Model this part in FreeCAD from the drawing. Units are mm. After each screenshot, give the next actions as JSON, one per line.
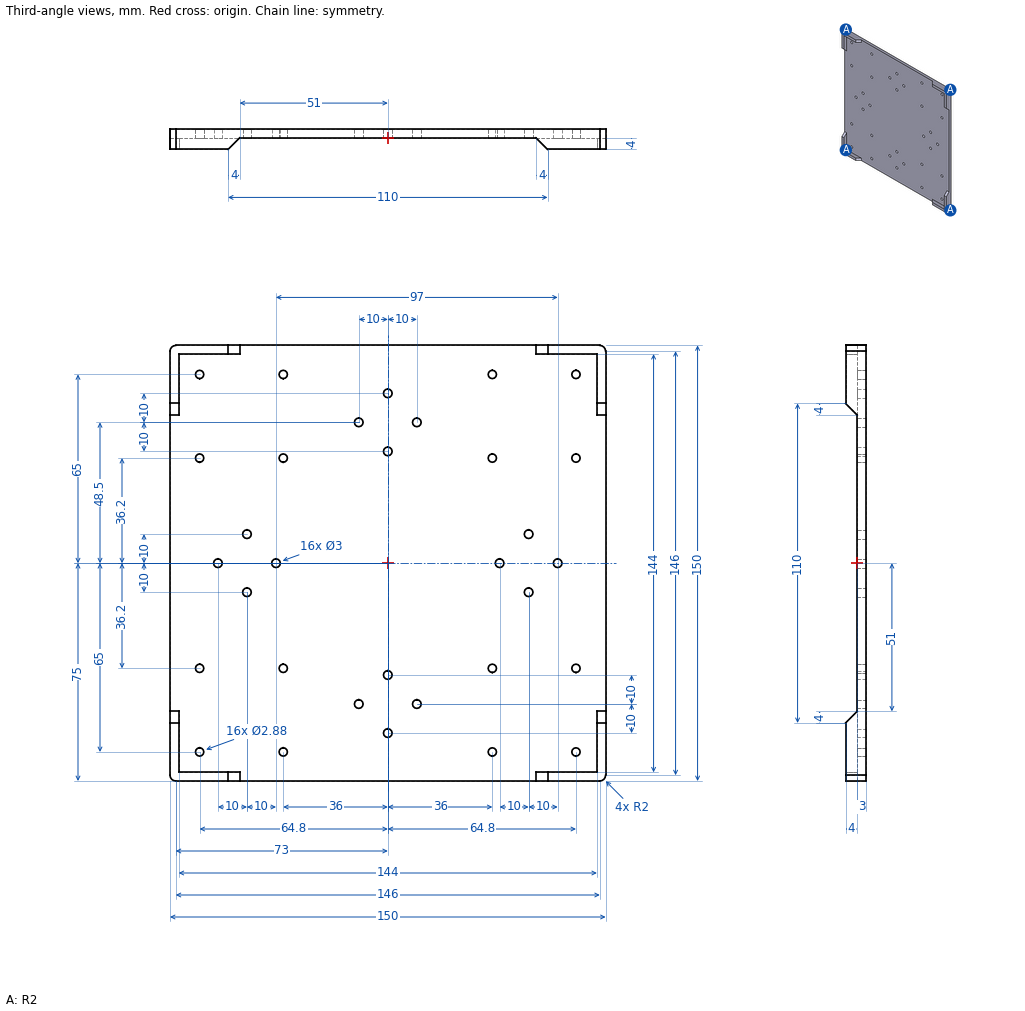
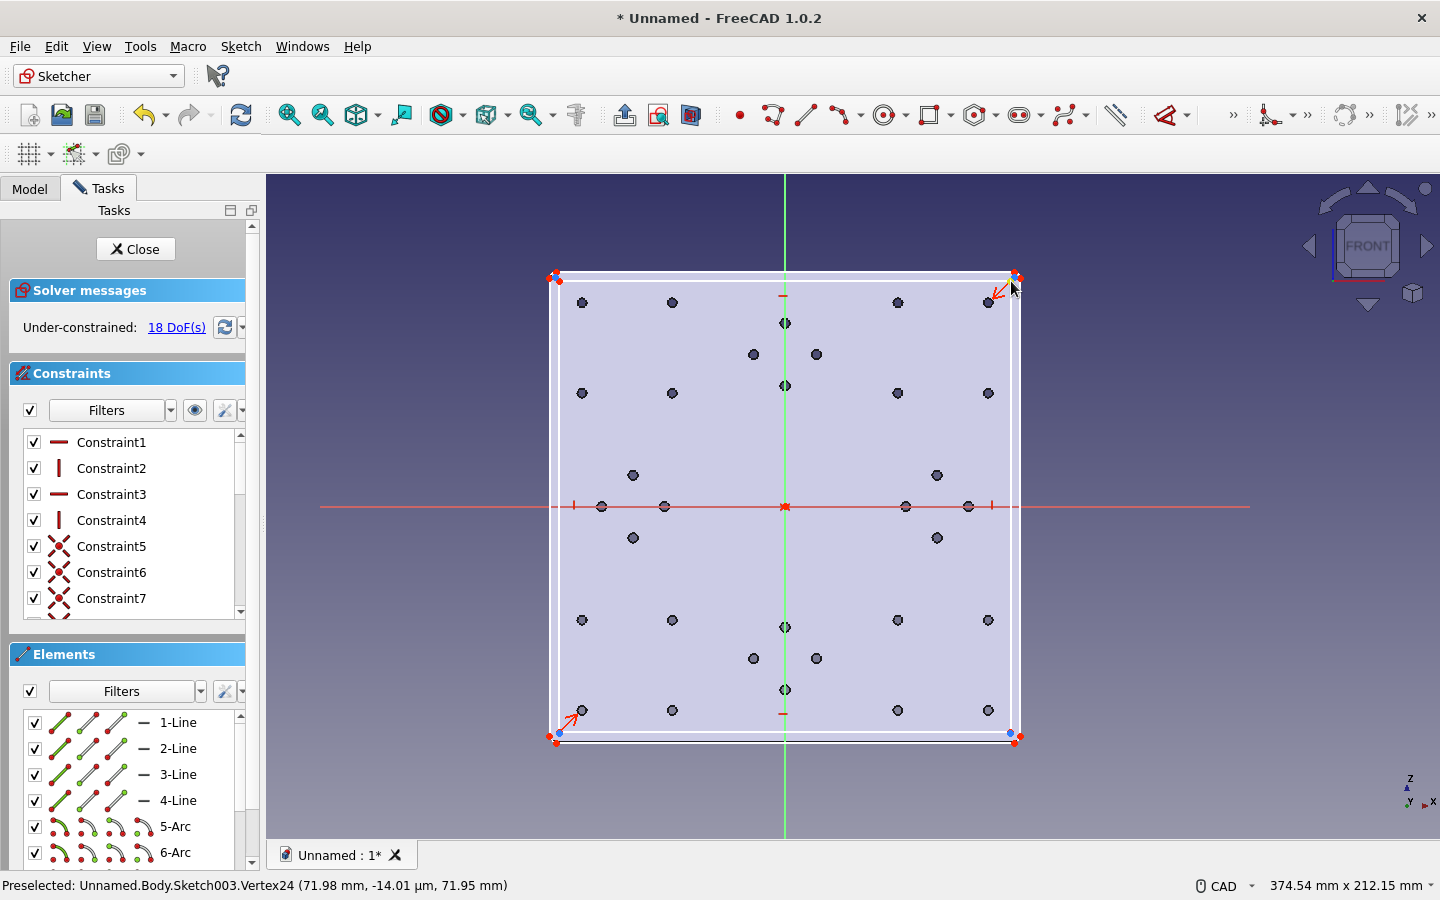
{"action": "scroll", "coordinate": [694, 743], "scroll_direction": "up", "scroll_amount": 2}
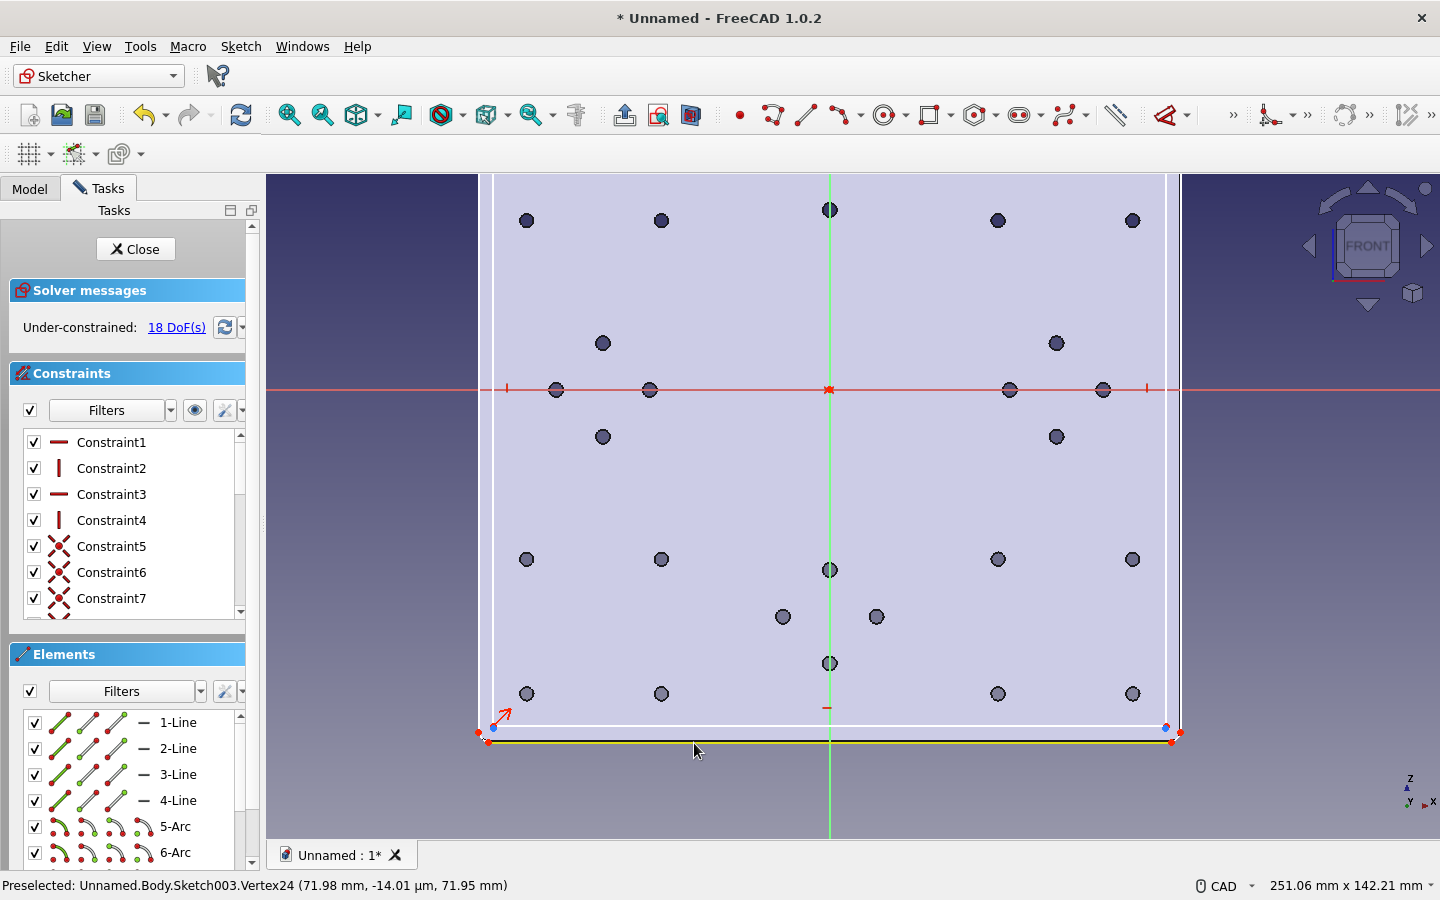
{"action": "left_click", "coordinate": [693, 743]}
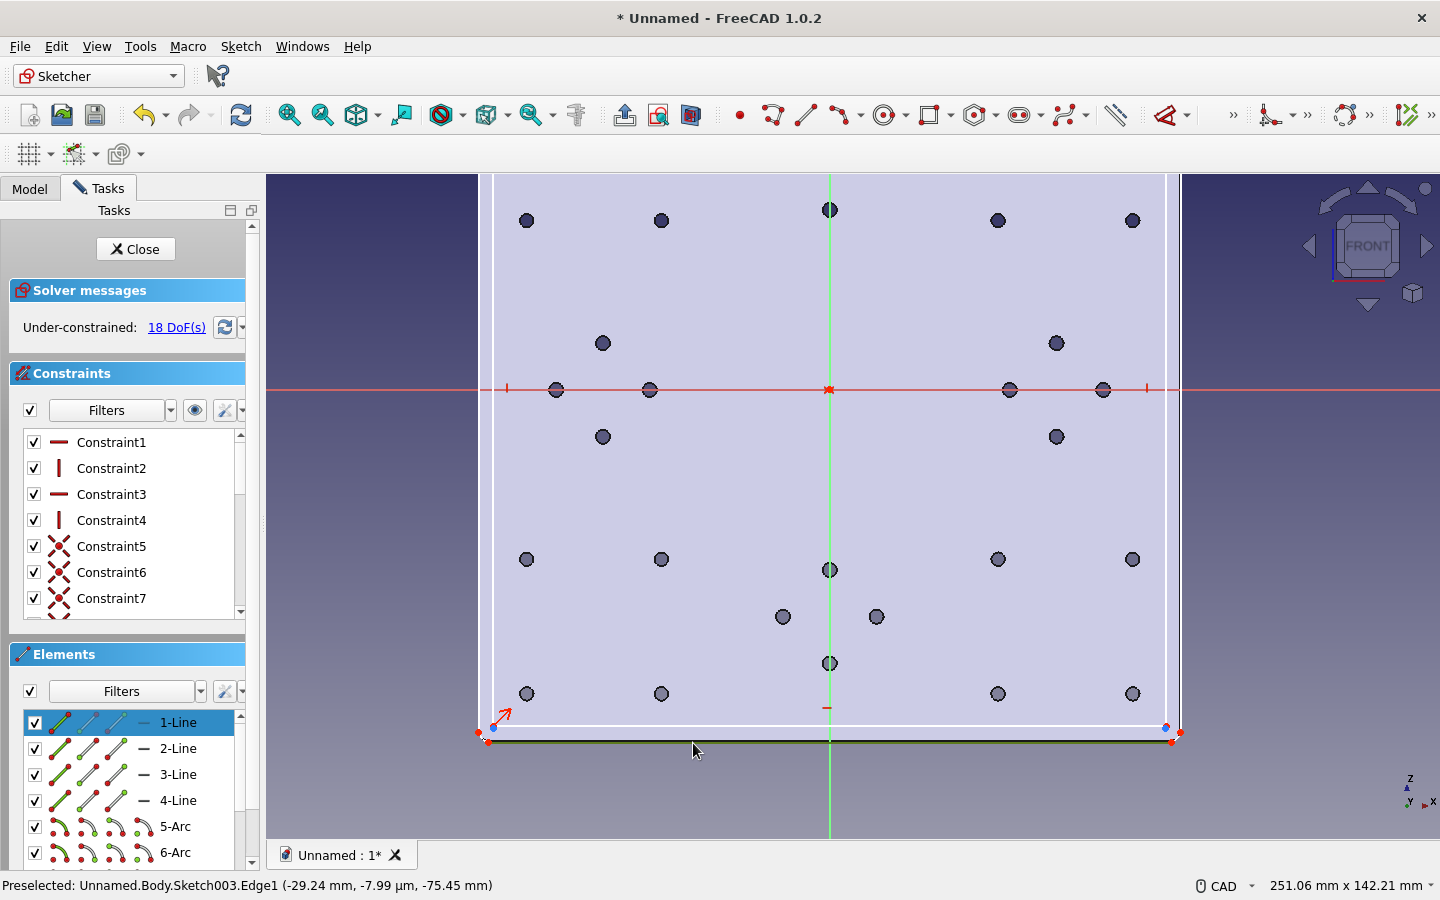
{"action": "scroll", "coordinate": [1177, 739], "scroll_direction": "up", "scroll_amount": 4}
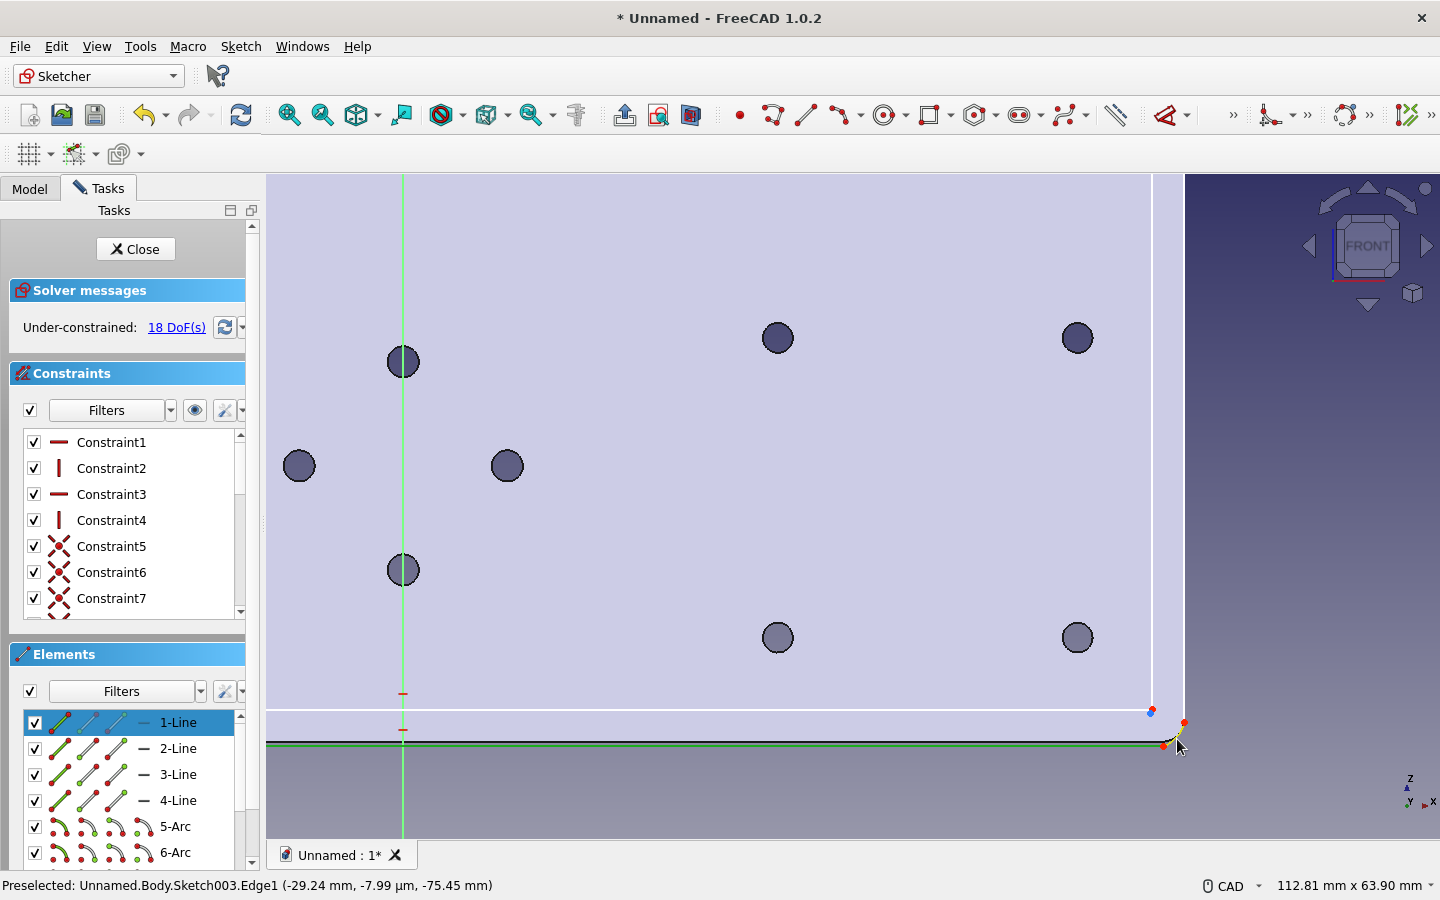
{"action": "left_click", "coordinate": [1177, 737]}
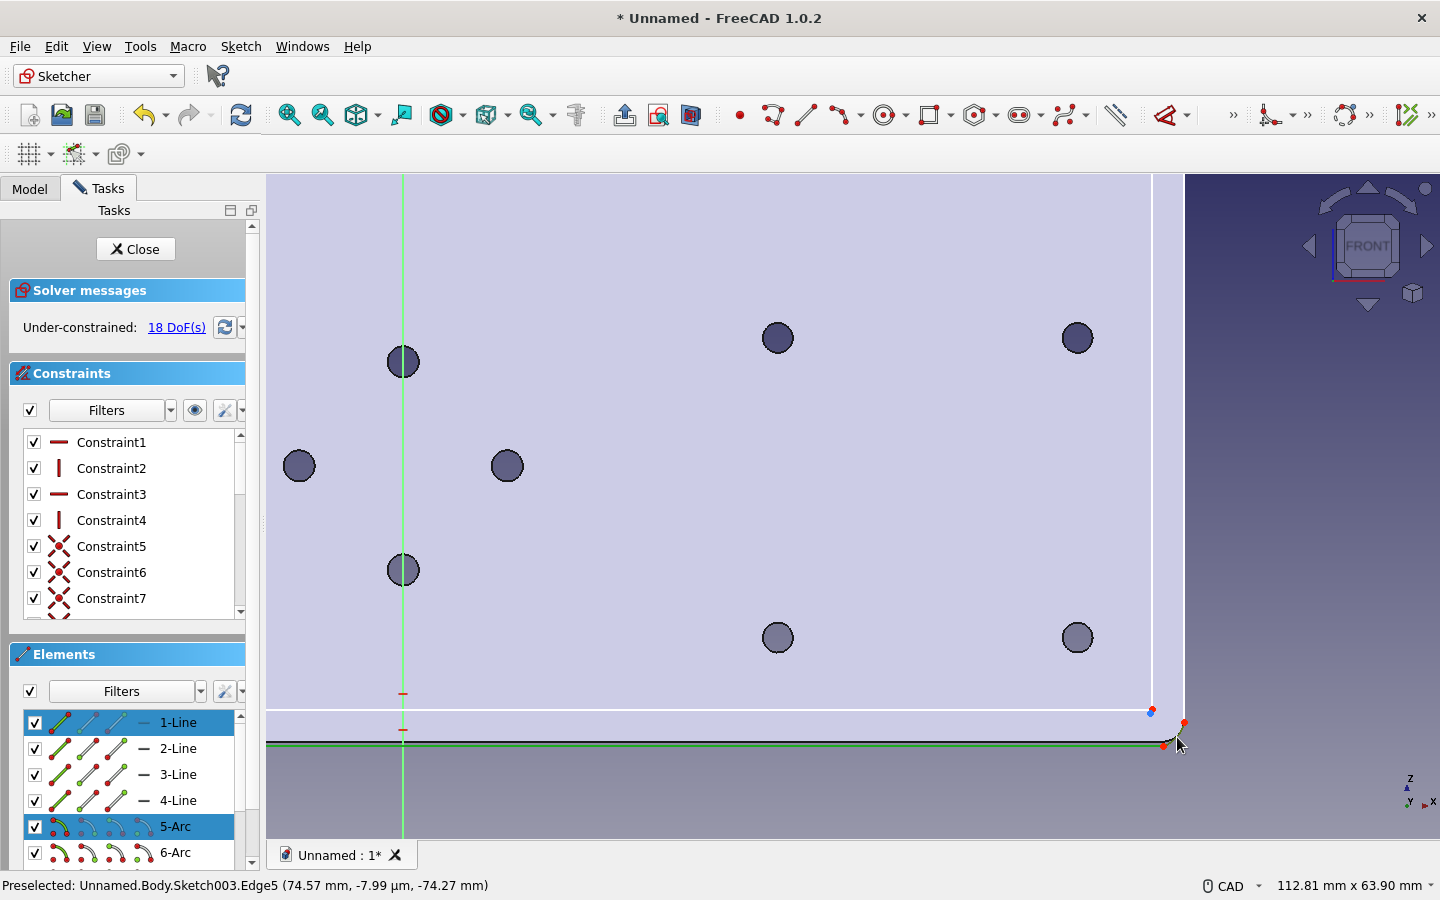
{"action": "key", "text": "t"}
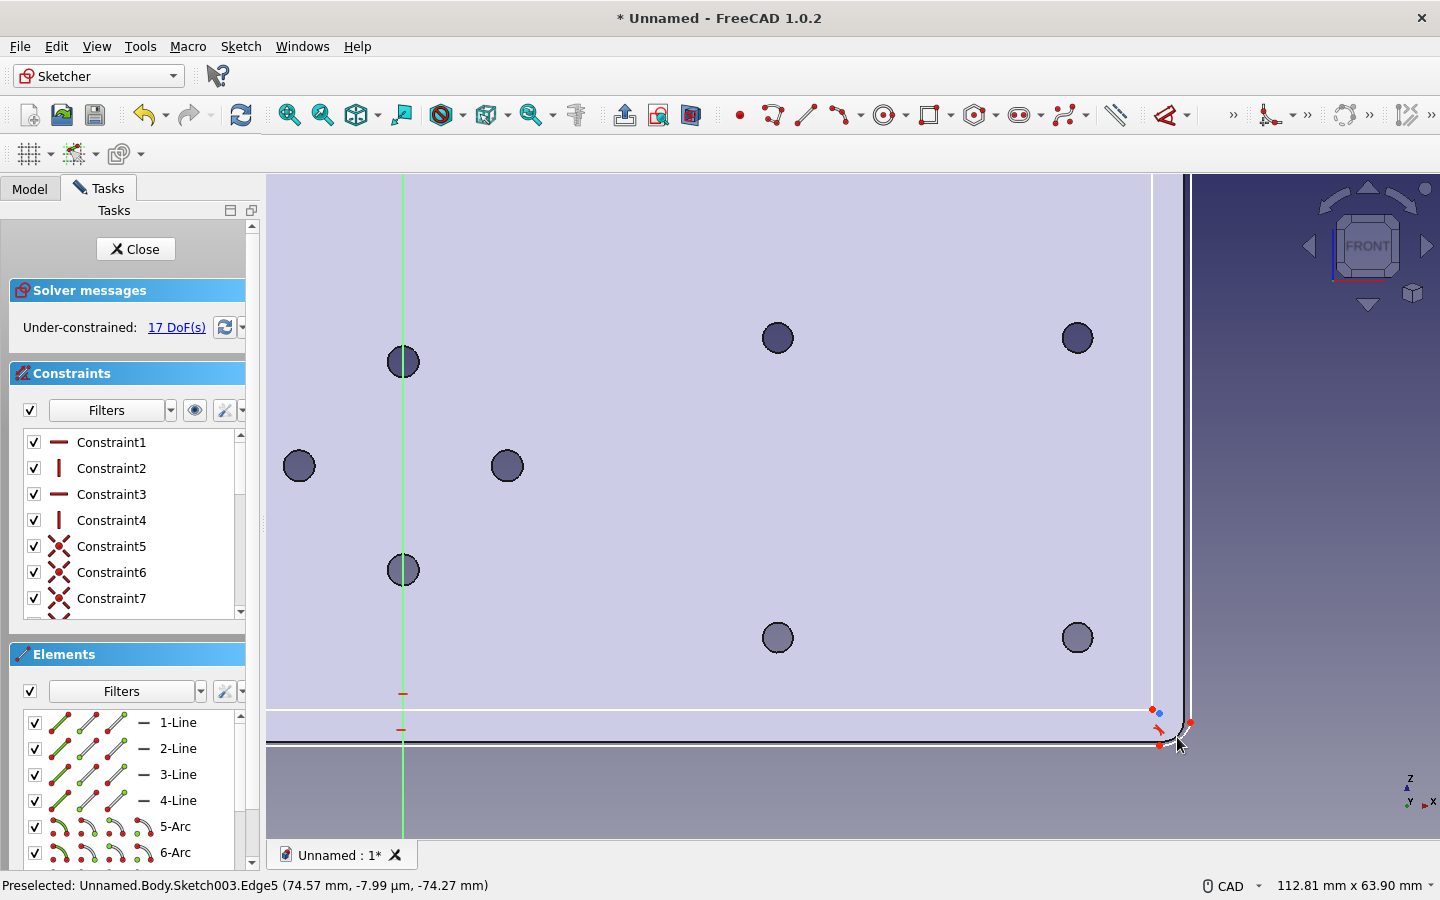
{"action": "left_click", "coordinate": [705, 746]}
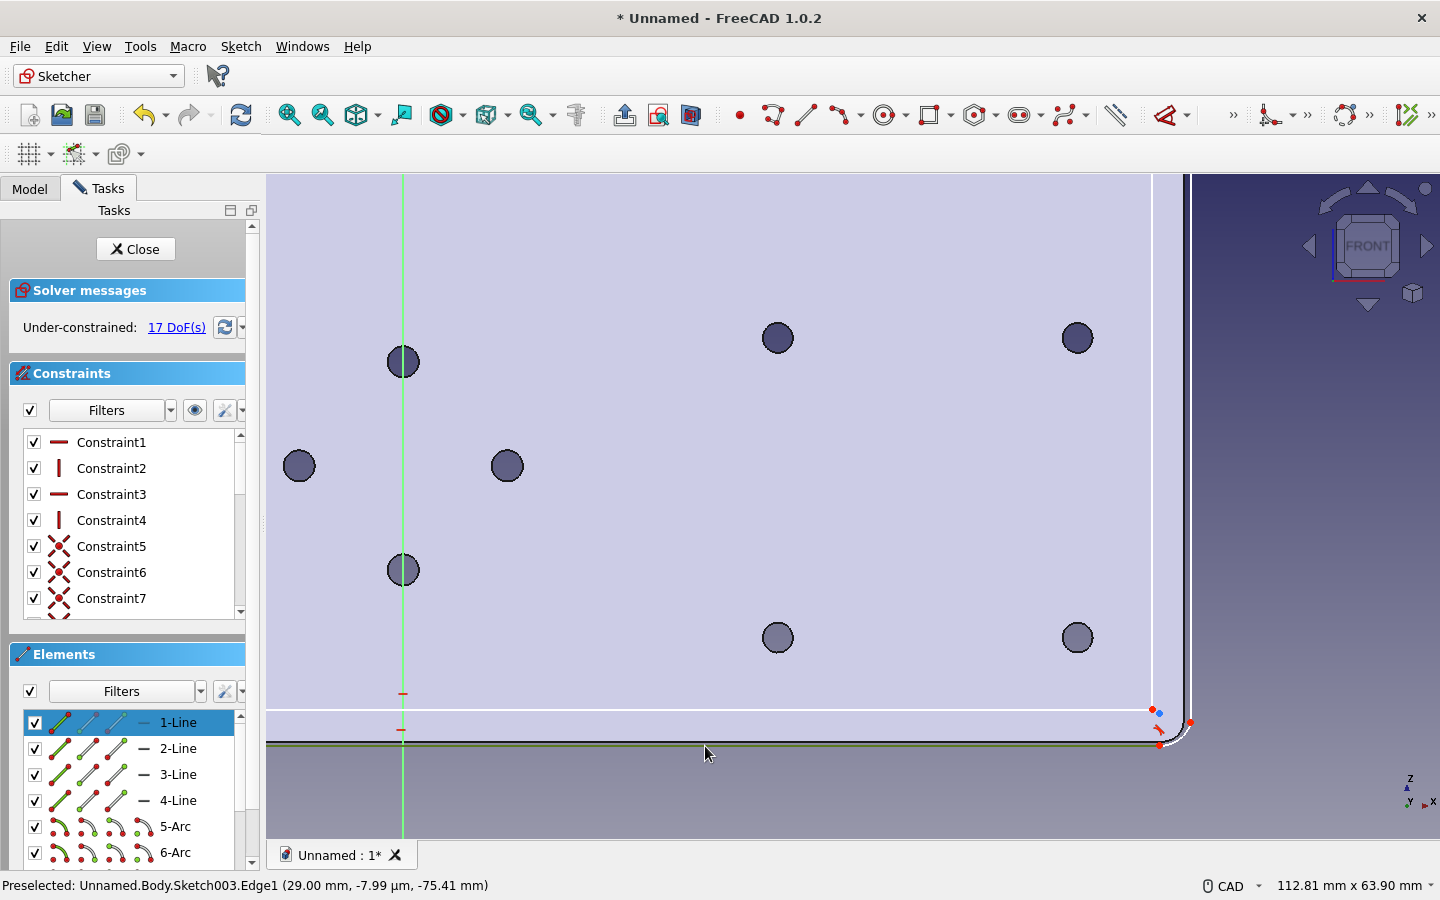
{"action": "scroll", "coordinate": [949, 742], "scroll_direction": "down", "scroll_amount": 6}